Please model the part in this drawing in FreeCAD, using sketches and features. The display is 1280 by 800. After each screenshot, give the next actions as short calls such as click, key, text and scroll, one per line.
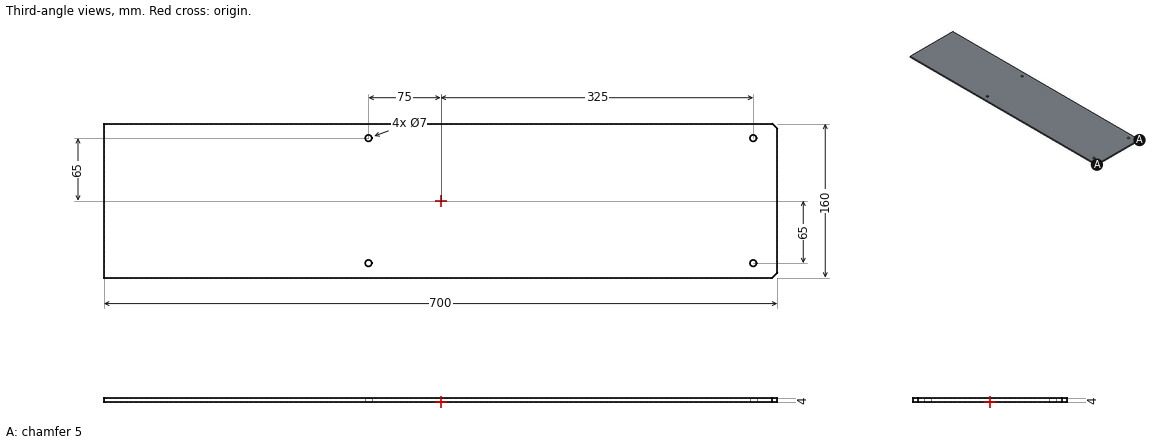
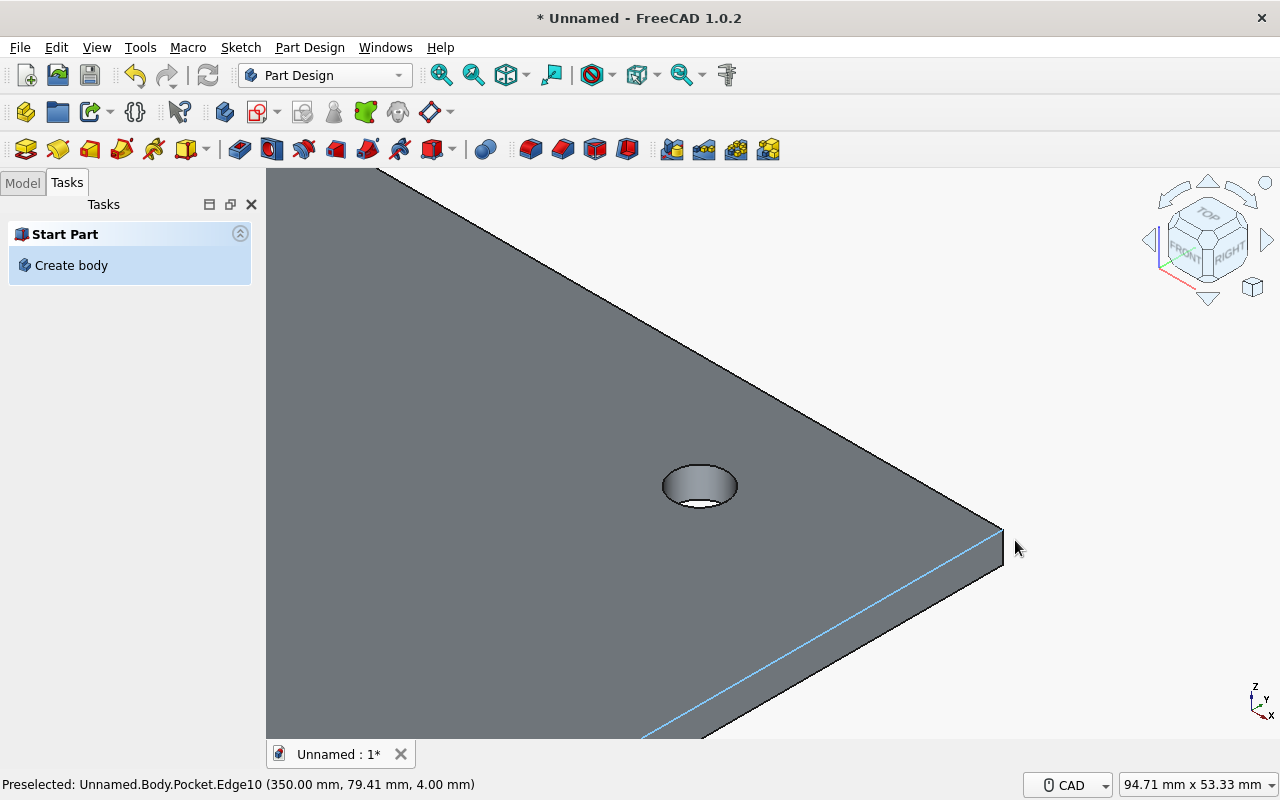
click(442, 76)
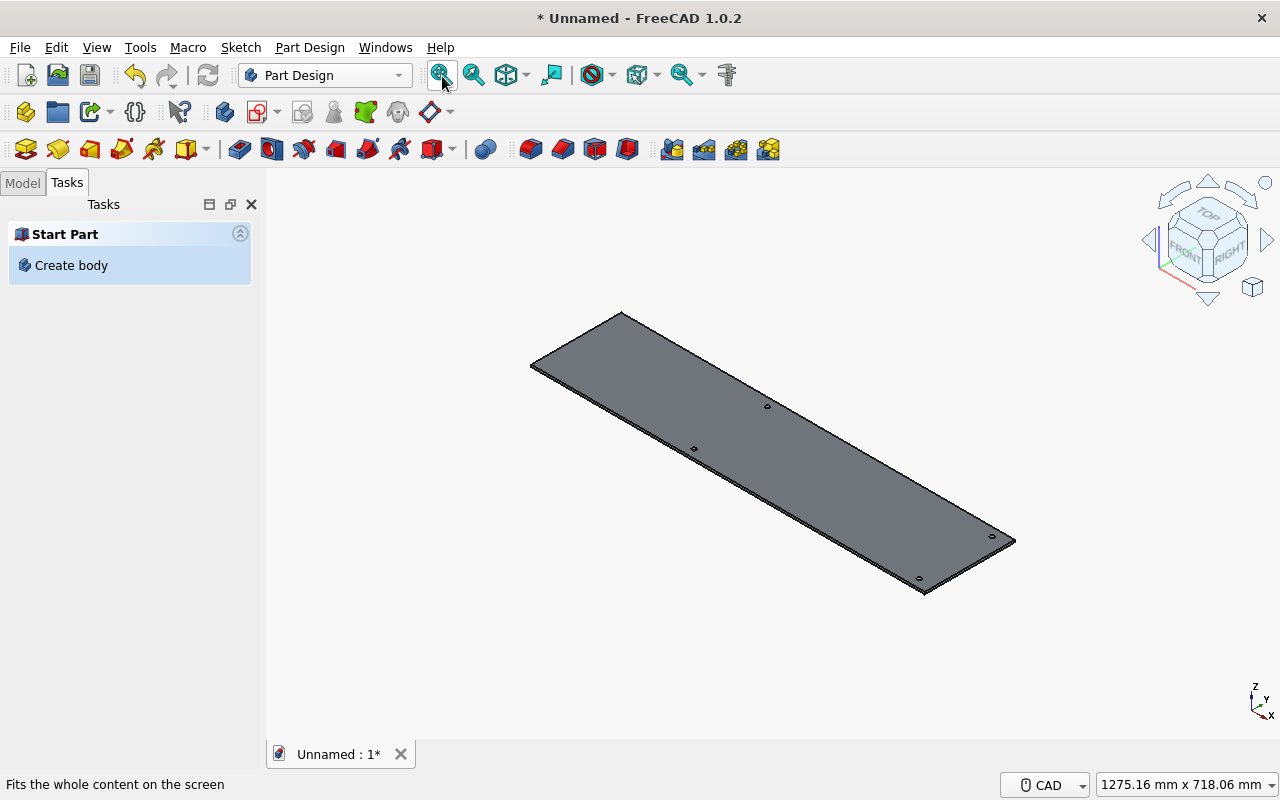
key(2)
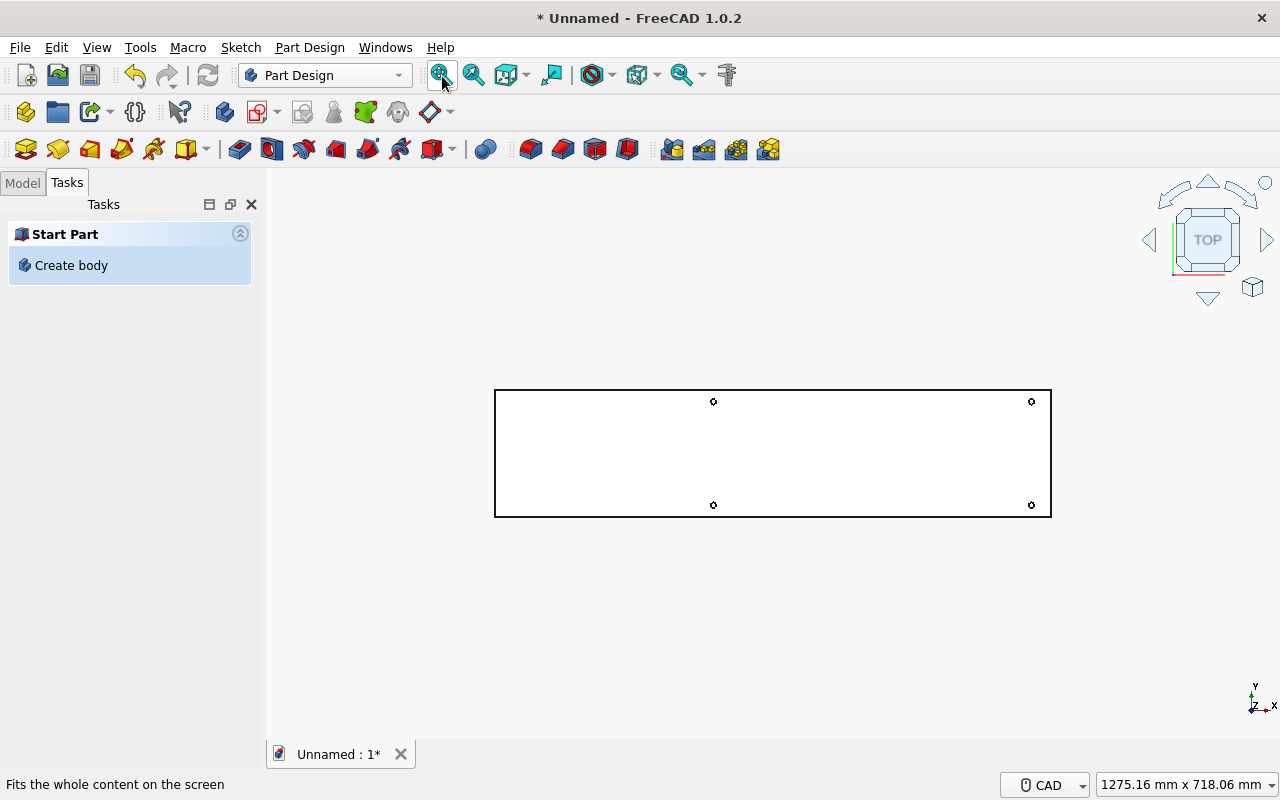
scroll(1051, 389, up, 13)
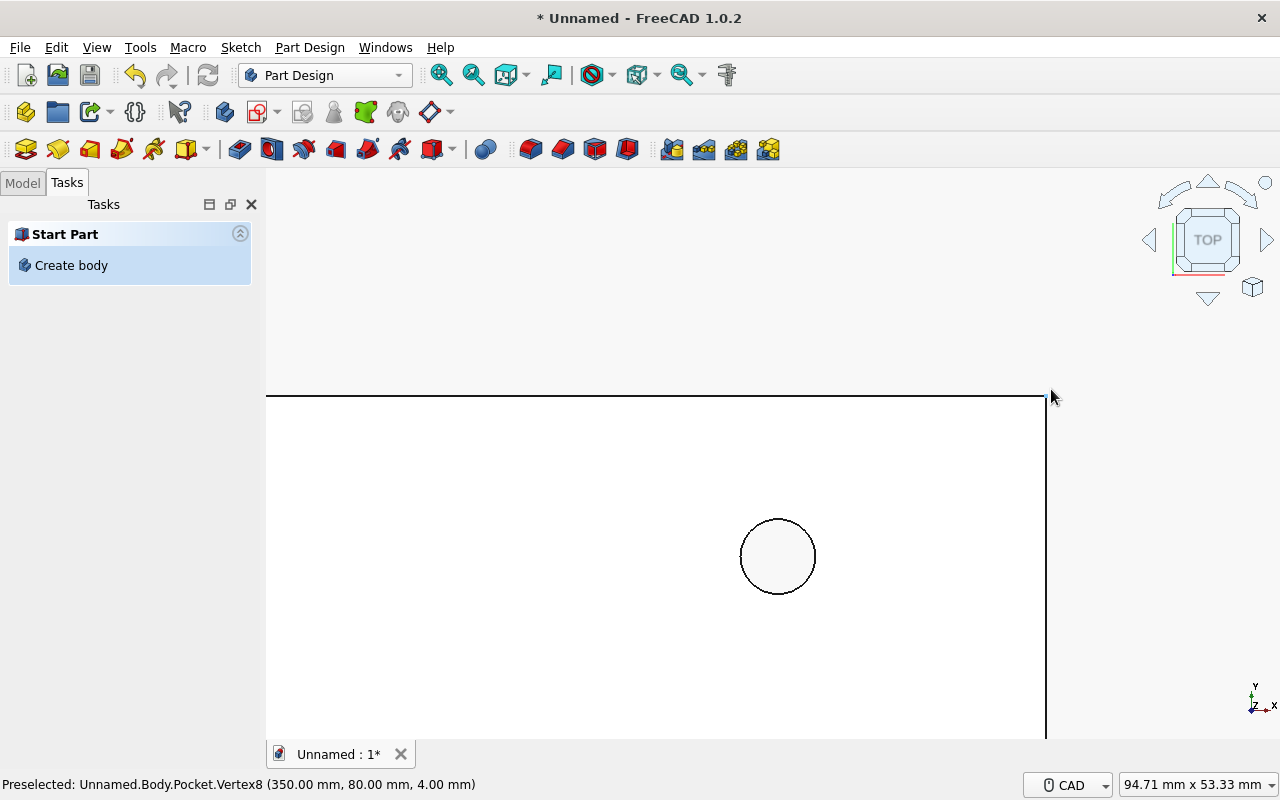
click(442, 76)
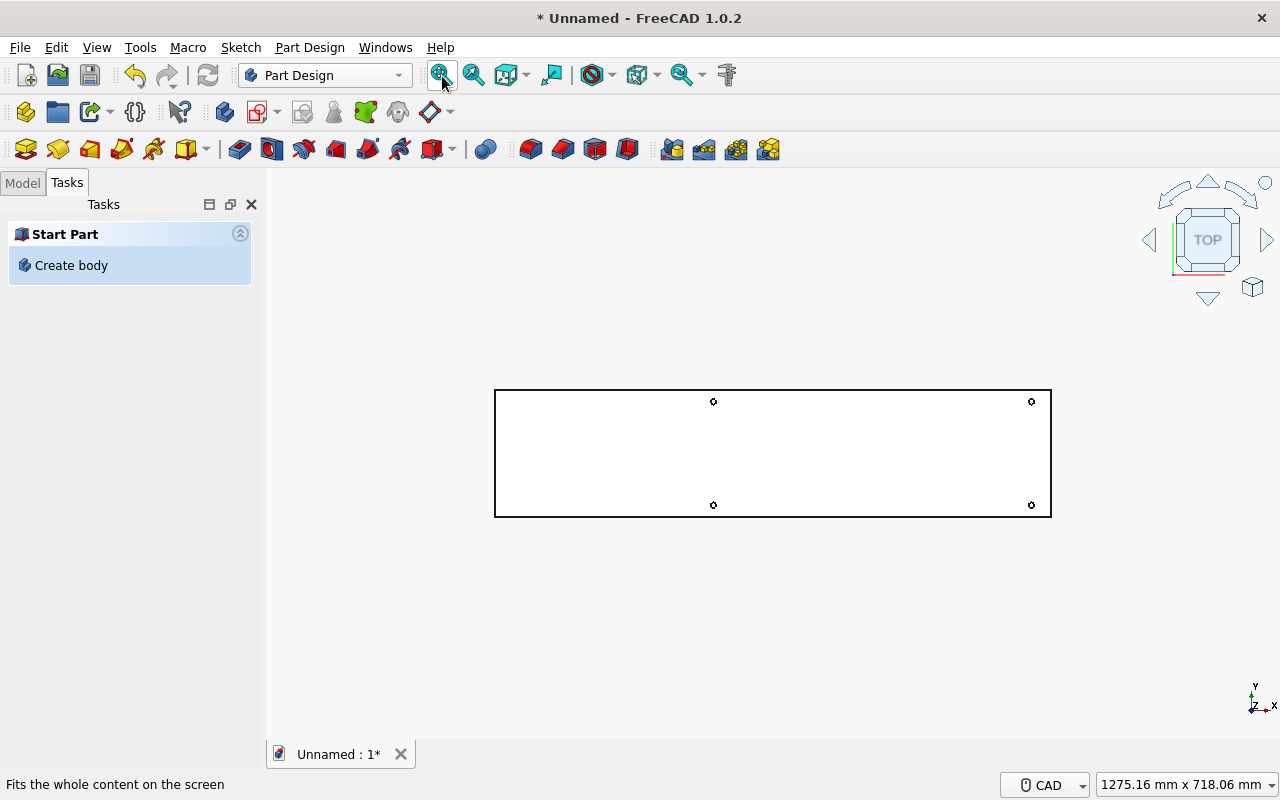
key(1)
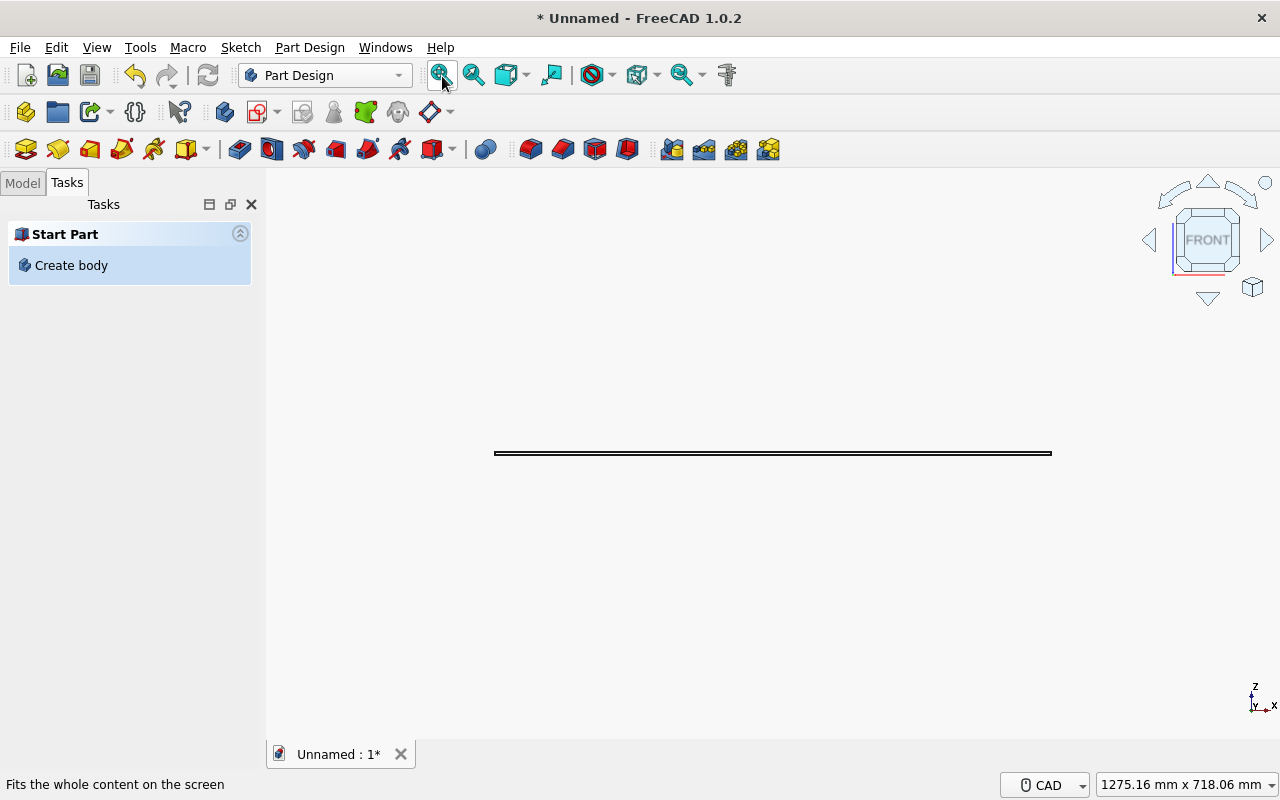
scroll(1051, 452, up, 13)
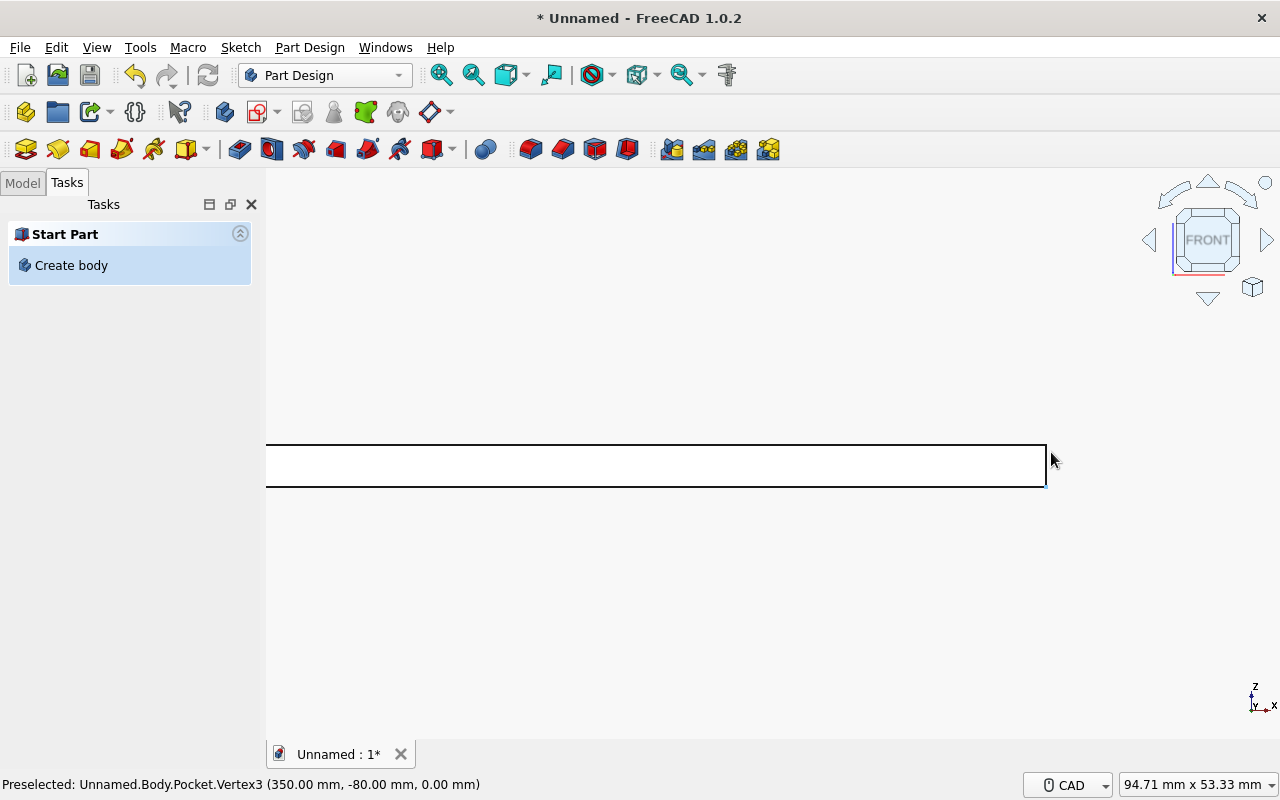
click(1046, 465)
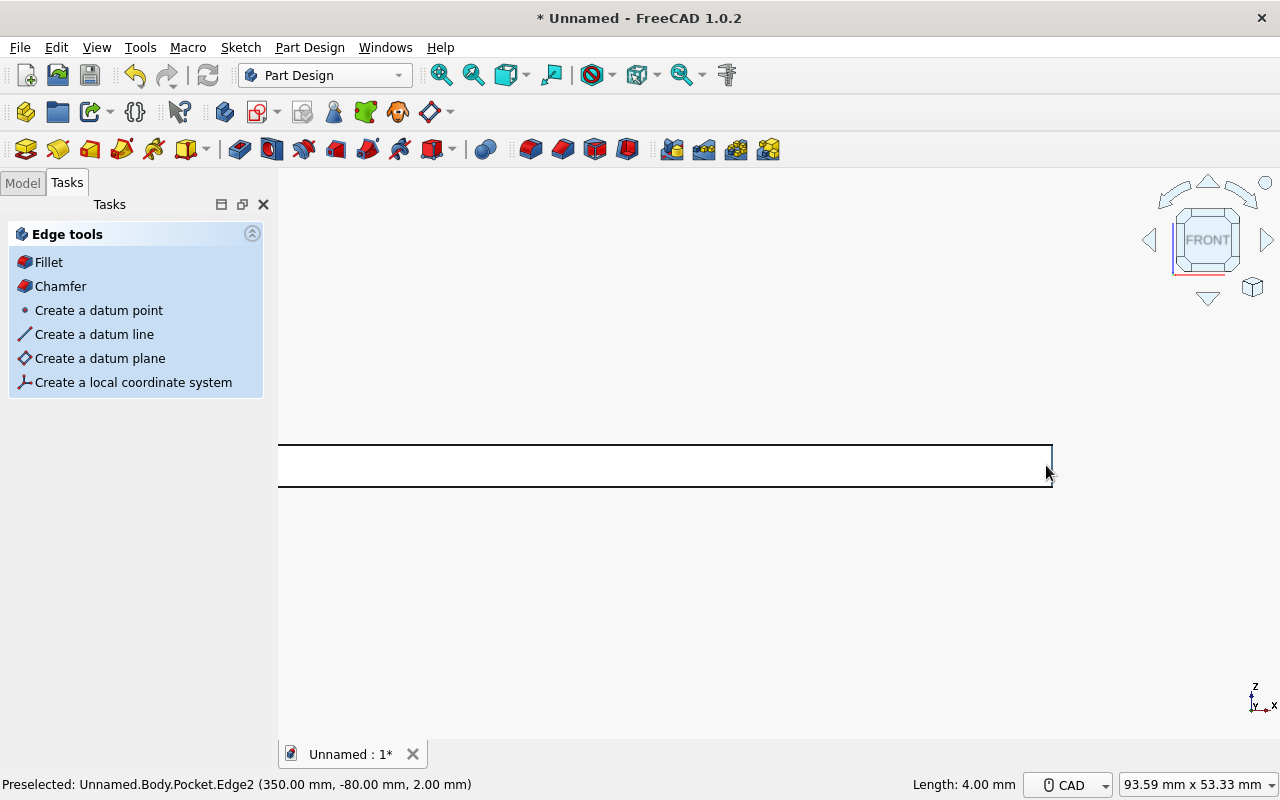
click(442, 76)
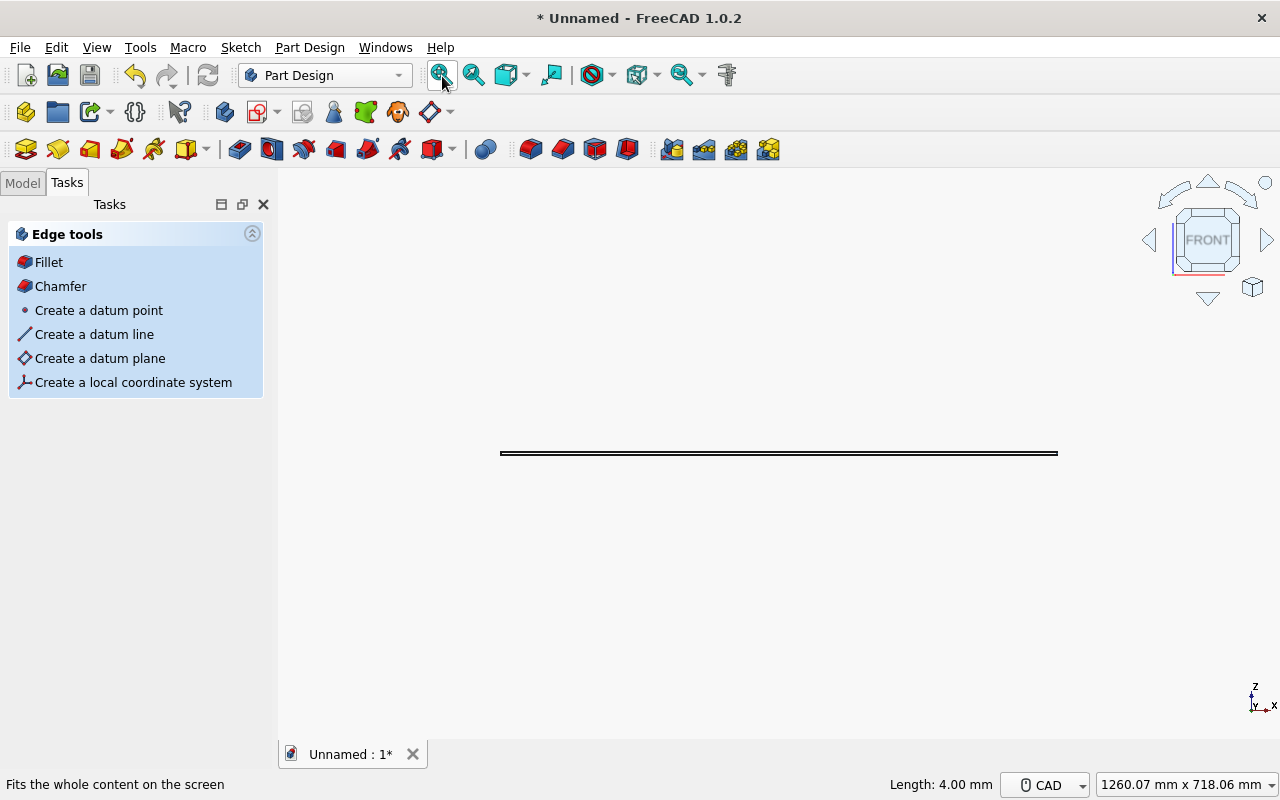
key(3)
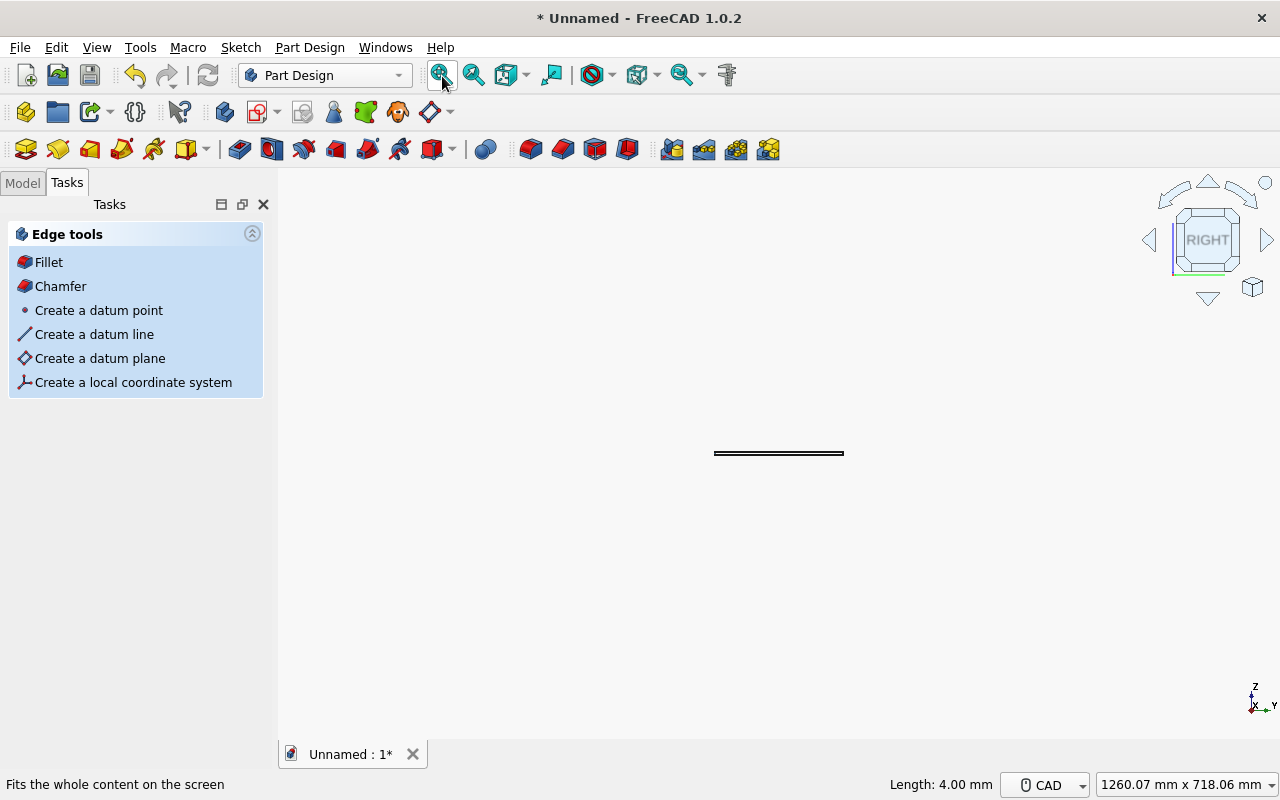
click(442, 76)